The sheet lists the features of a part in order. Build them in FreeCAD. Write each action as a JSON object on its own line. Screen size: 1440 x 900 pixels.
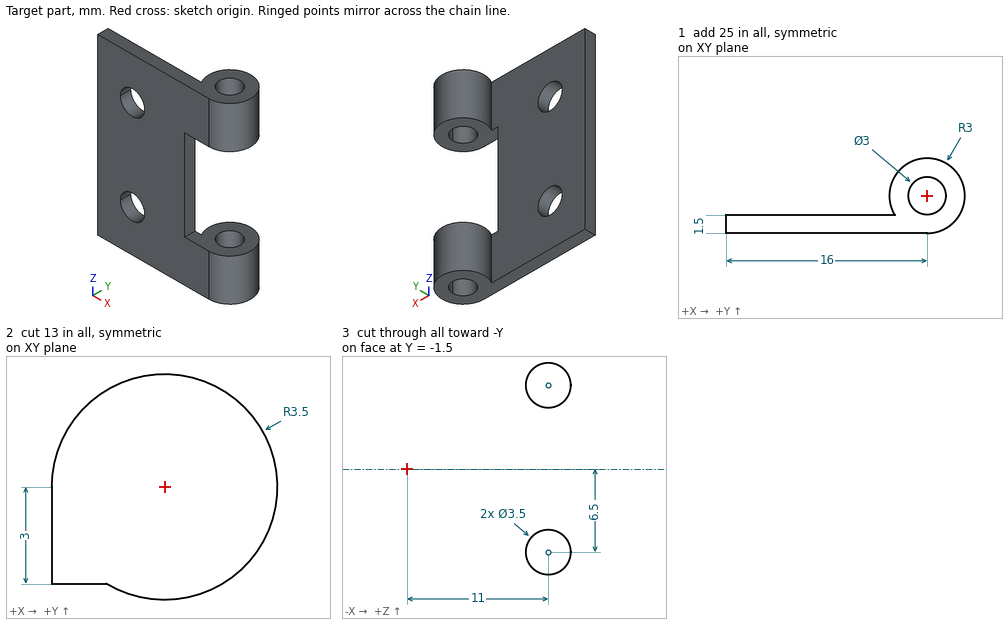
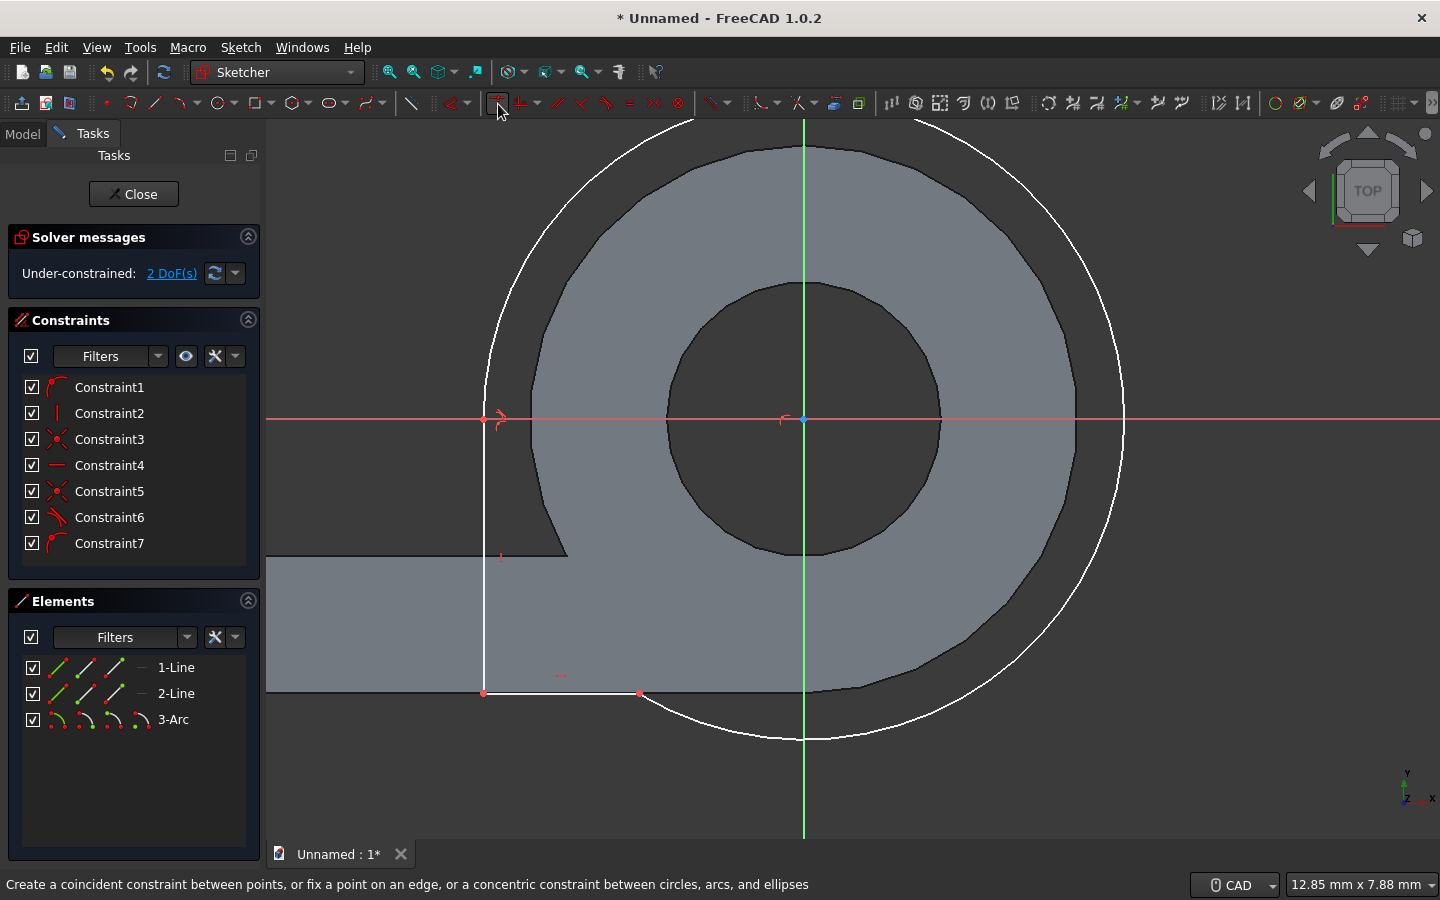
{"action": "left_click", "coordinate": [450, 104]}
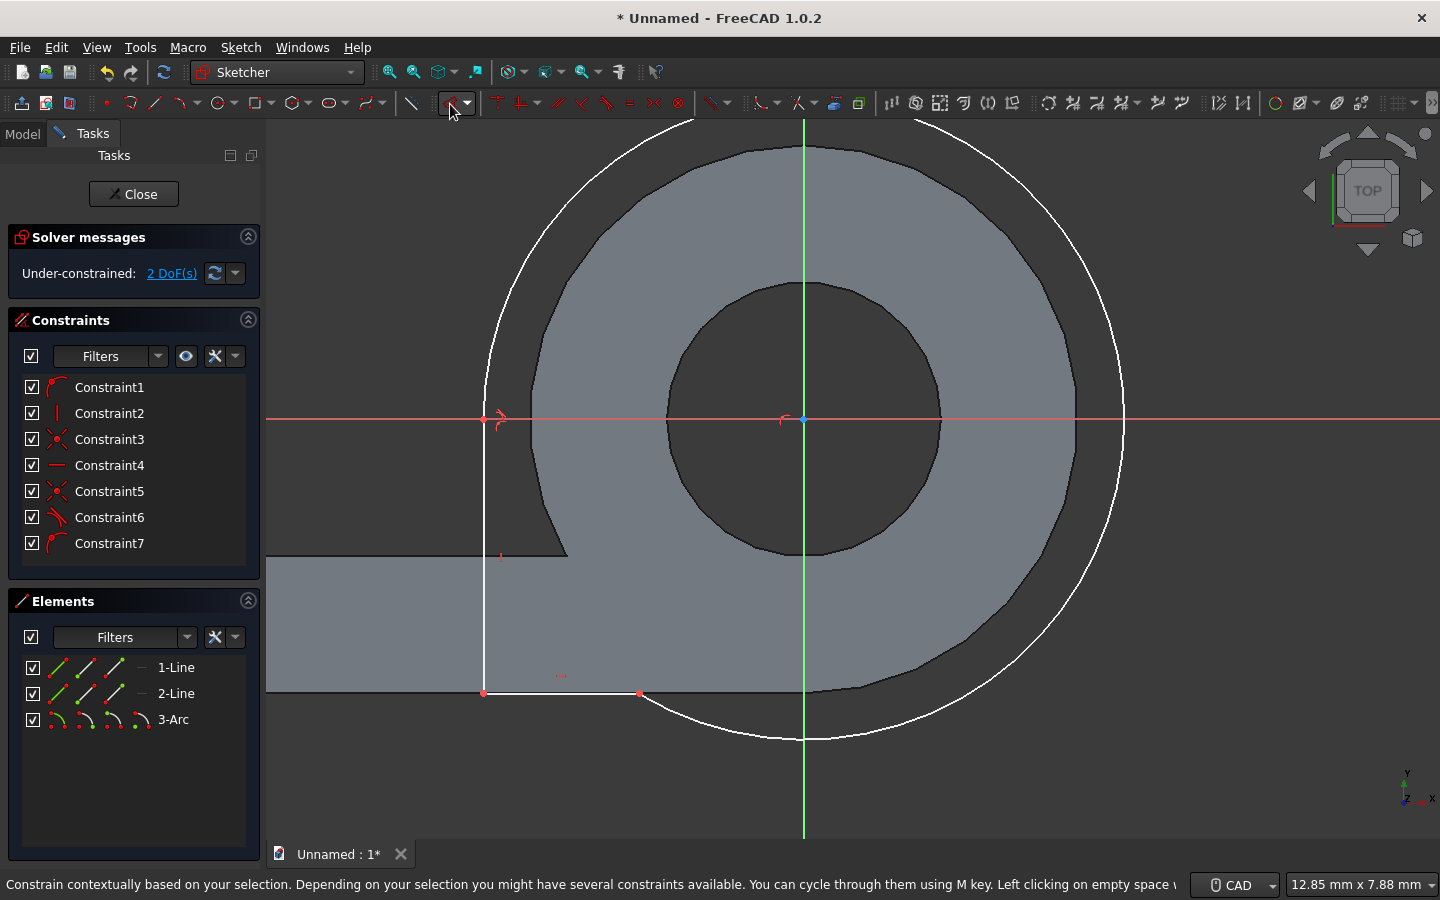
{"action": "left_click", "coordinate": [1079, 583]}
{"action": "left_click", "coordinate": [1107, 599]}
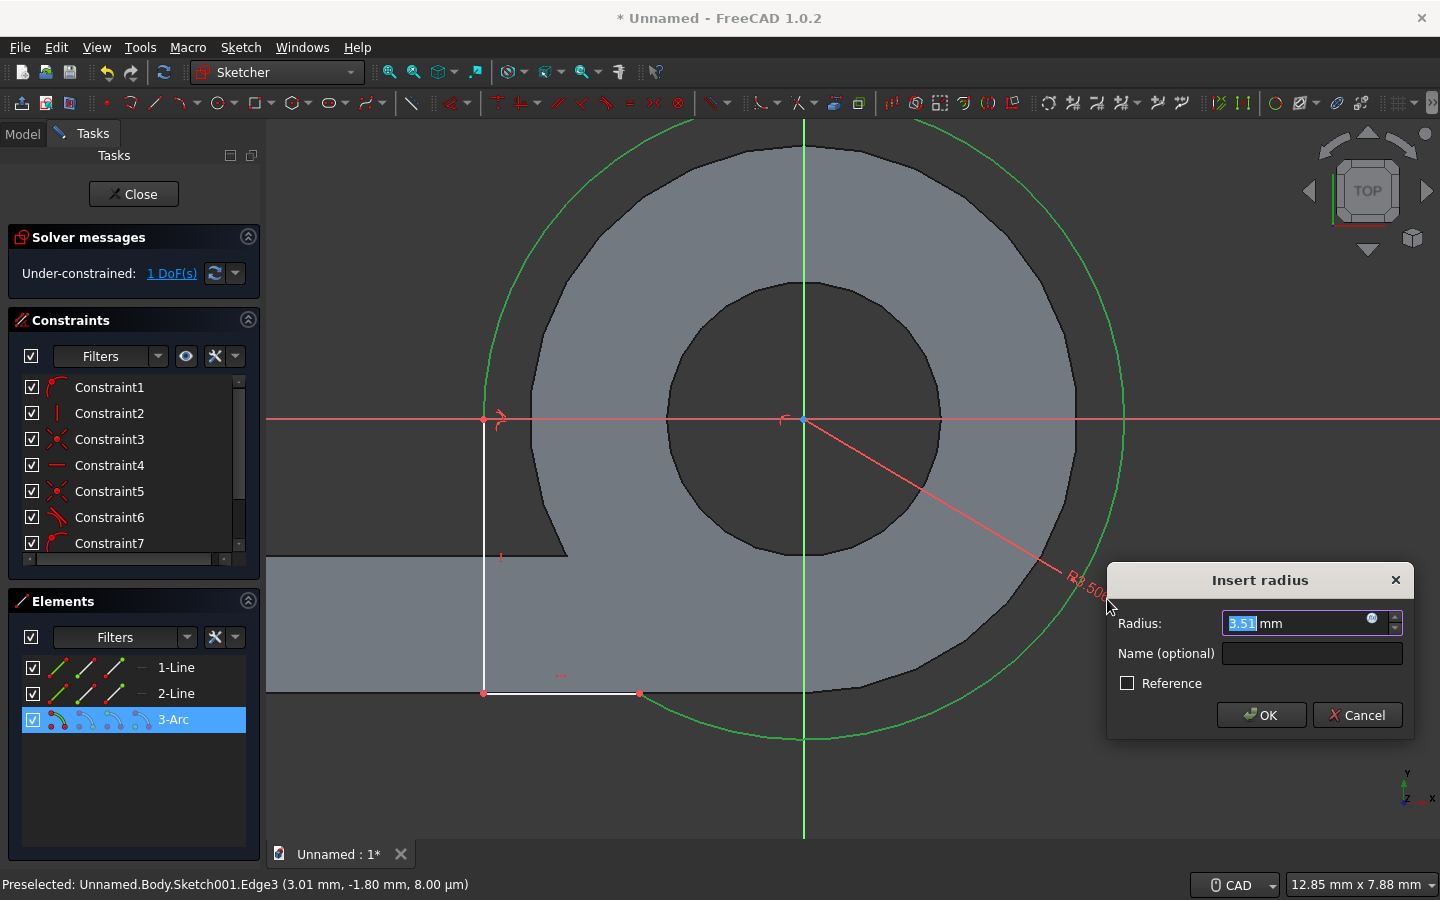
{"action": "type", "text": "3.5"}
{"action": "key", "text": "Return"}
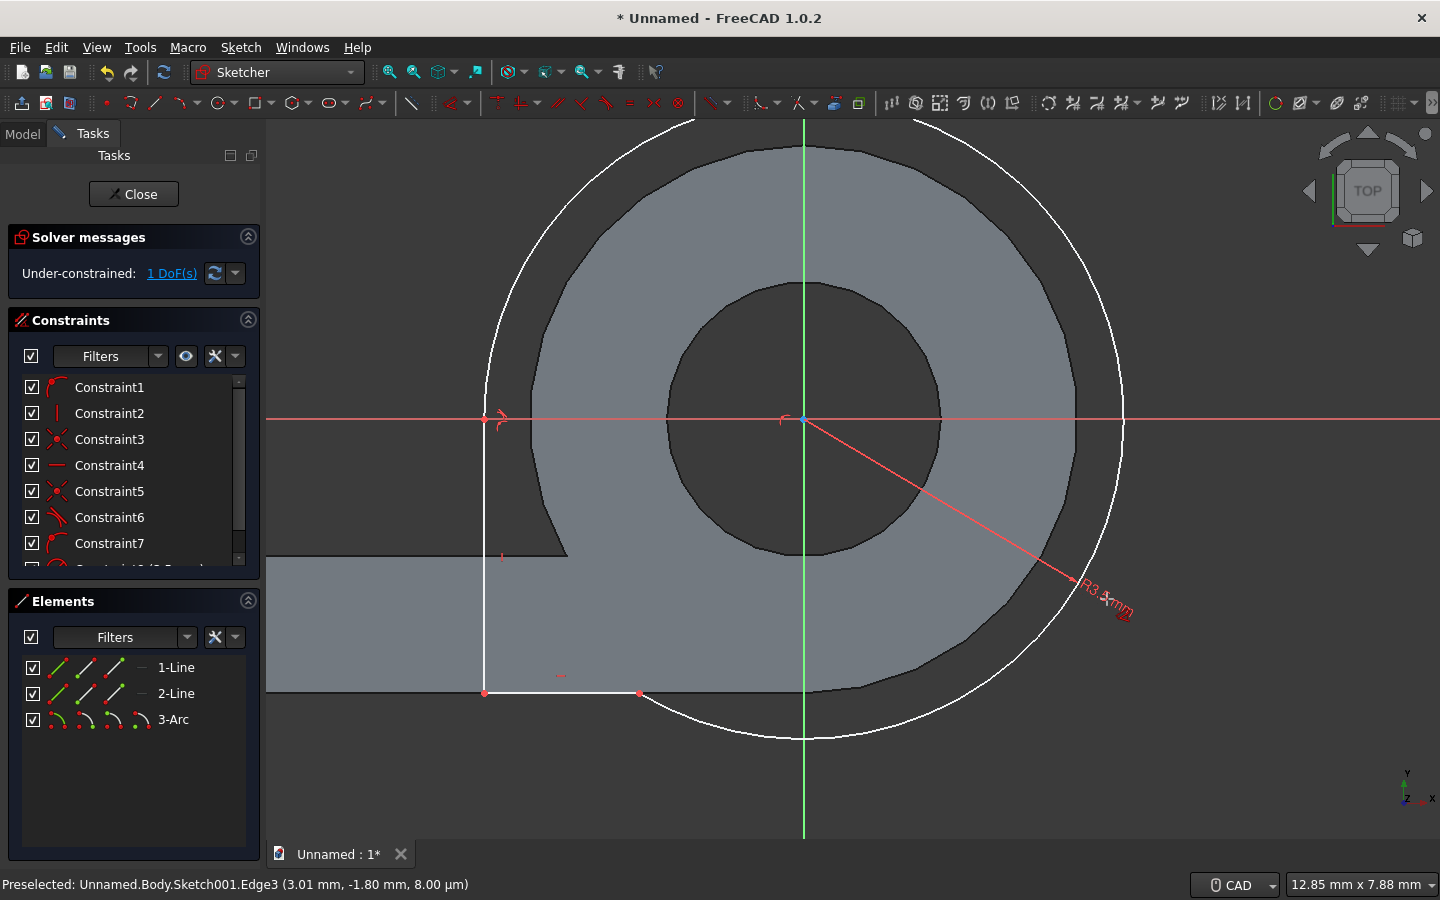
{"action": "left_click", "coordinate": [484, 502]}
{"action": "left_click", "coordinate": [450, 556]}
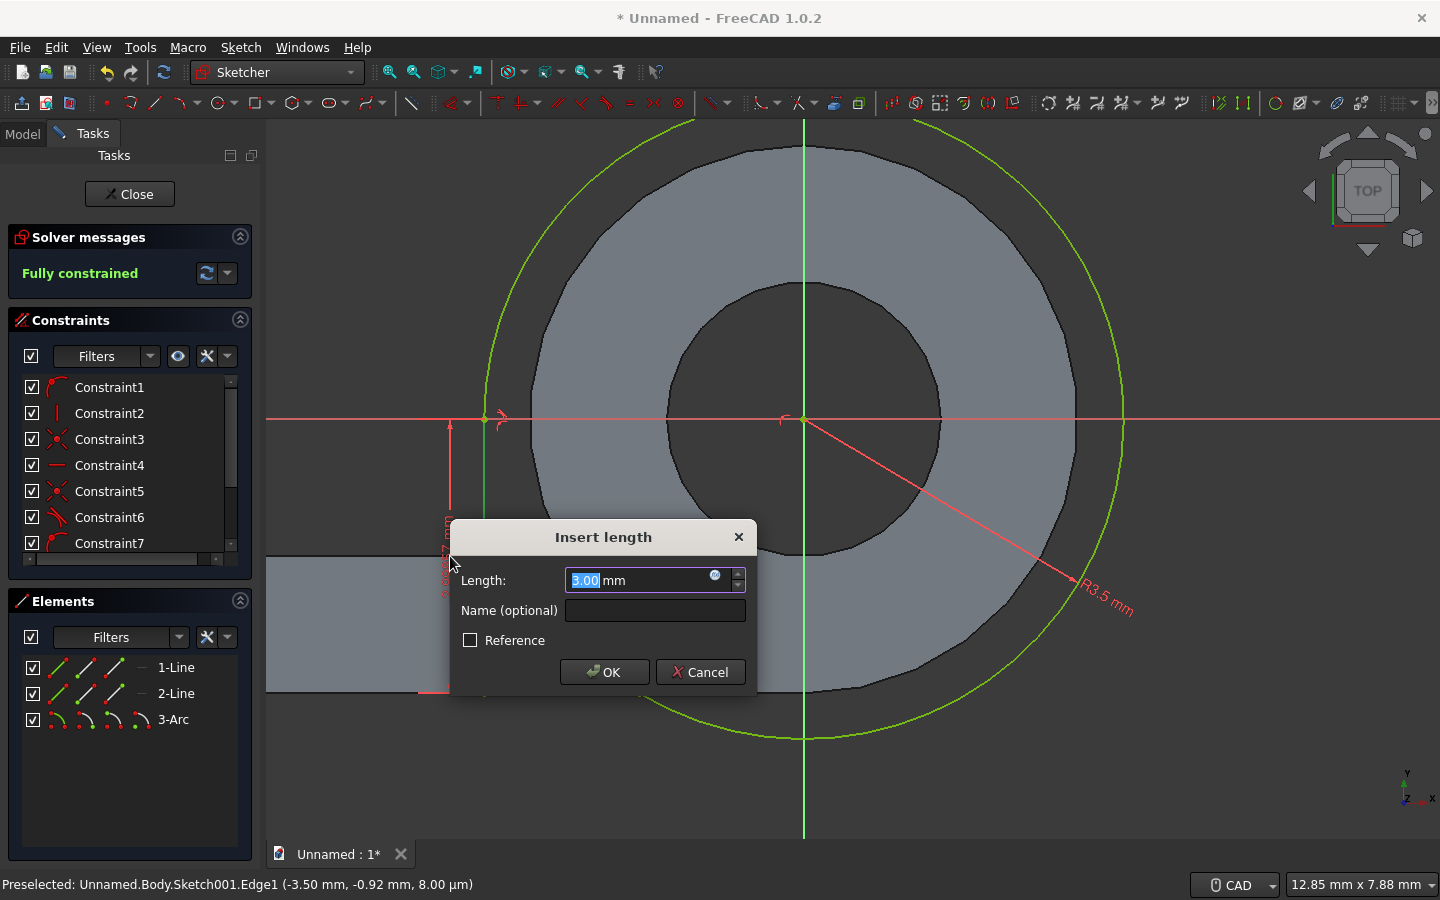
{"action": "type", "text": "3"}
{"action": "key", "text": "Return"}
{"action": "key", "text": "Escape"}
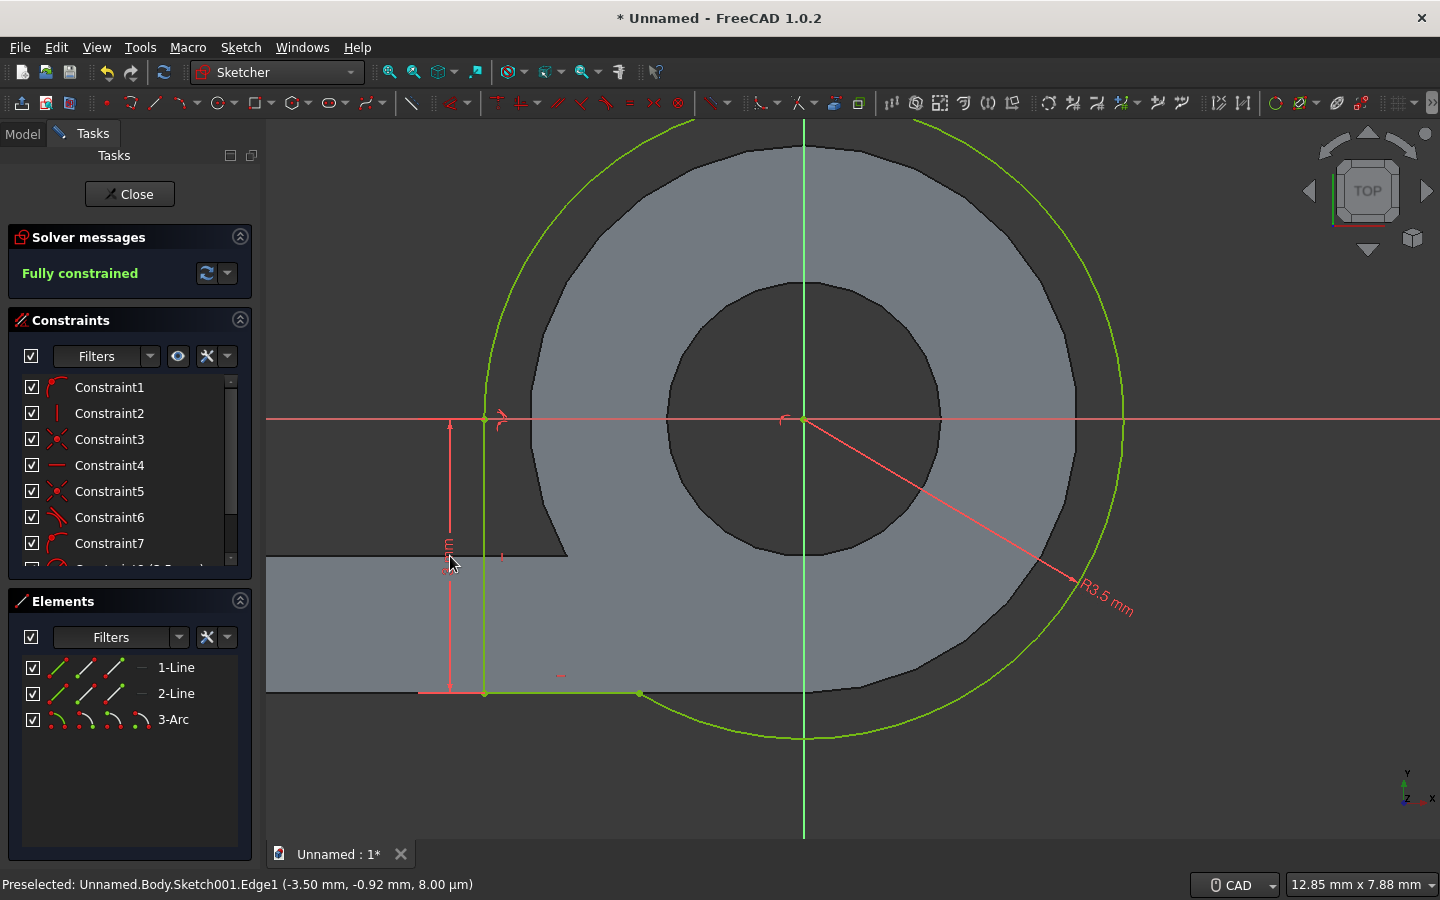
{"action": "left_click", "coordinate": [130, 194]}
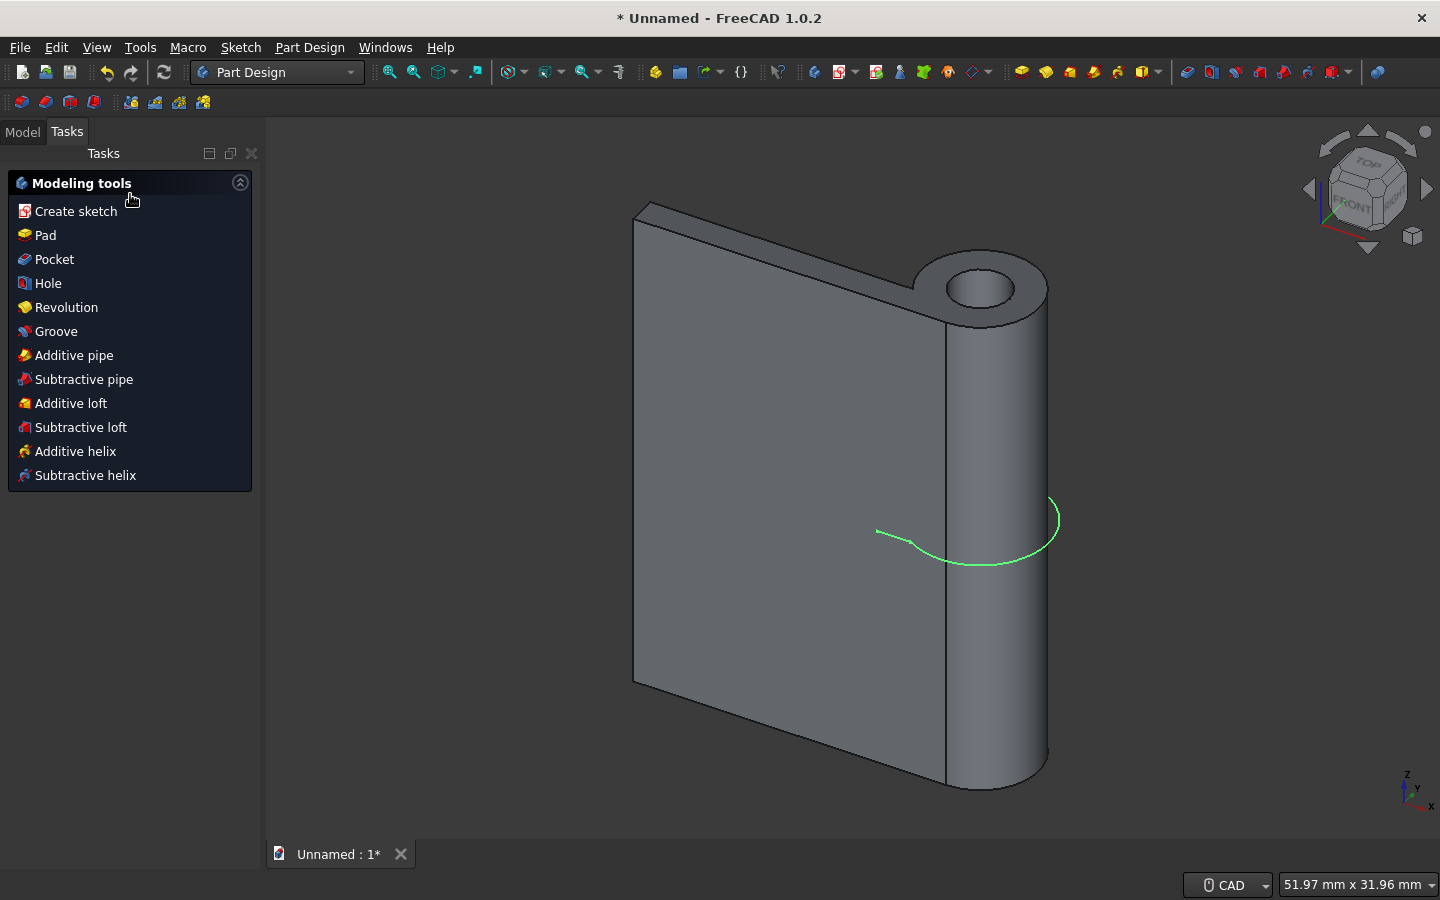
{"action": "left_click", "coordinate": [1188, 72]}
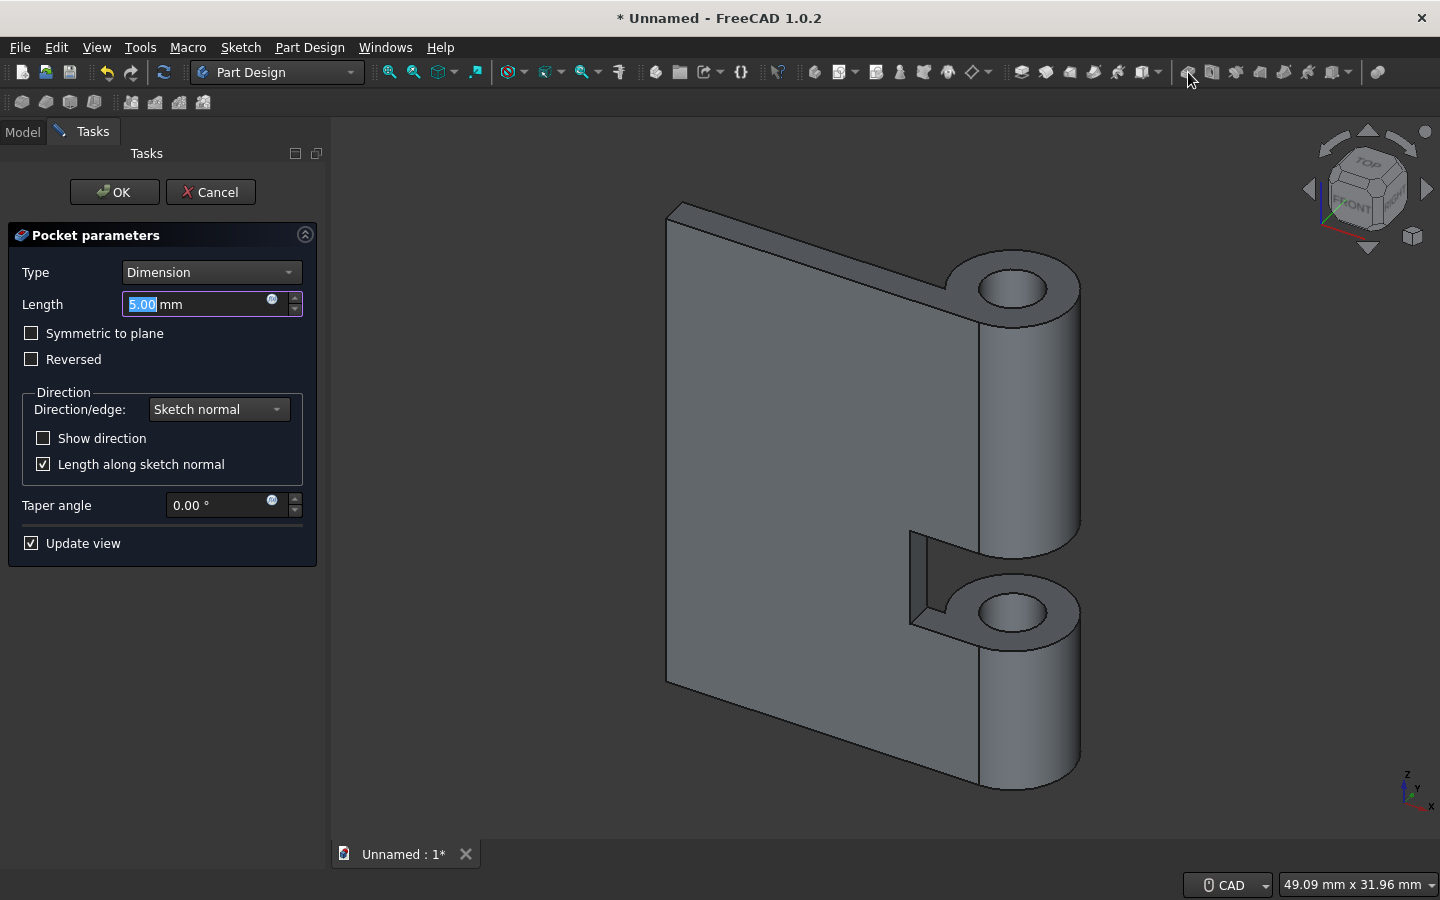
{"action": "type", "text": "13"}
{"action": "key", "text": "Tab"}